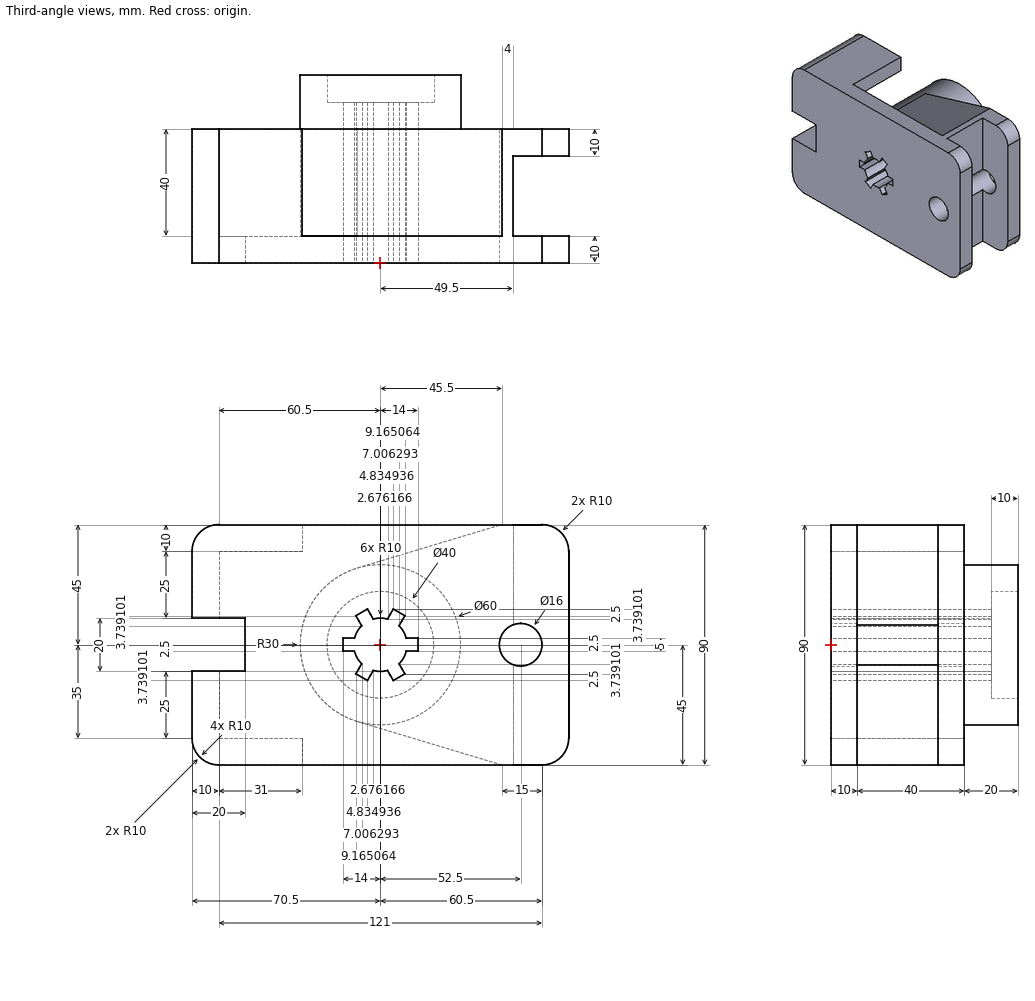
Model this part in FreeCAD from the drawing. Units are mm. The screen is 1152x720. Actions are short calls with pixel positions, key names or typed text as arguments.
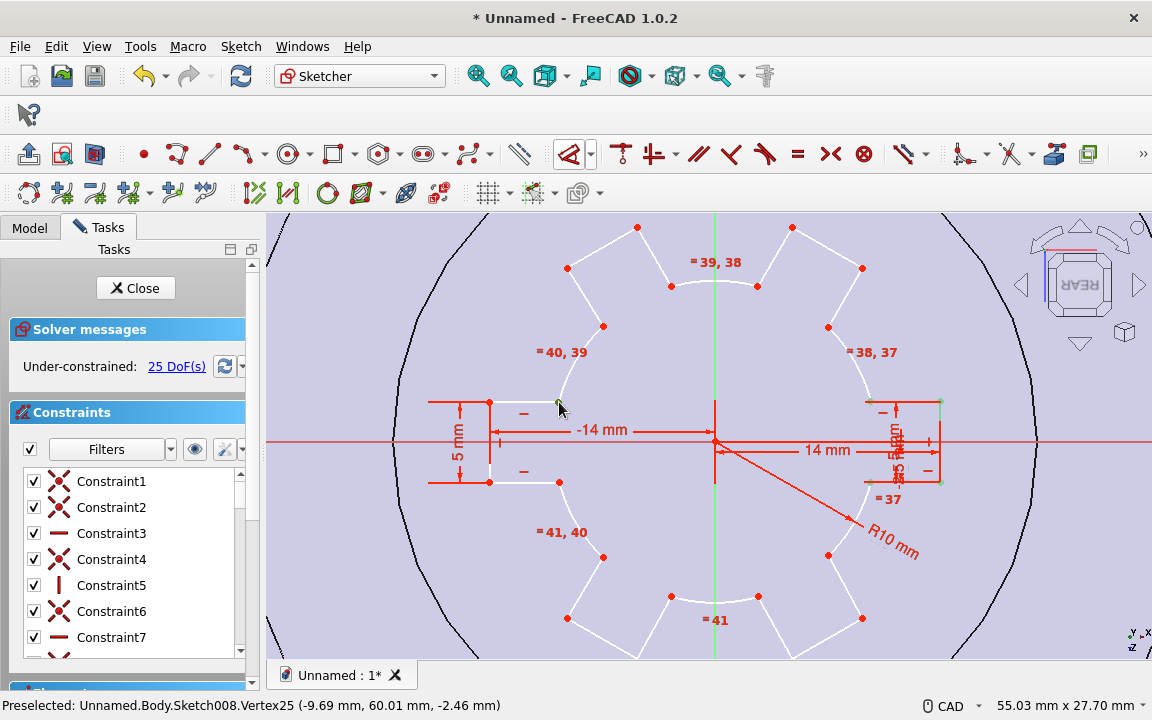
click(590, 154)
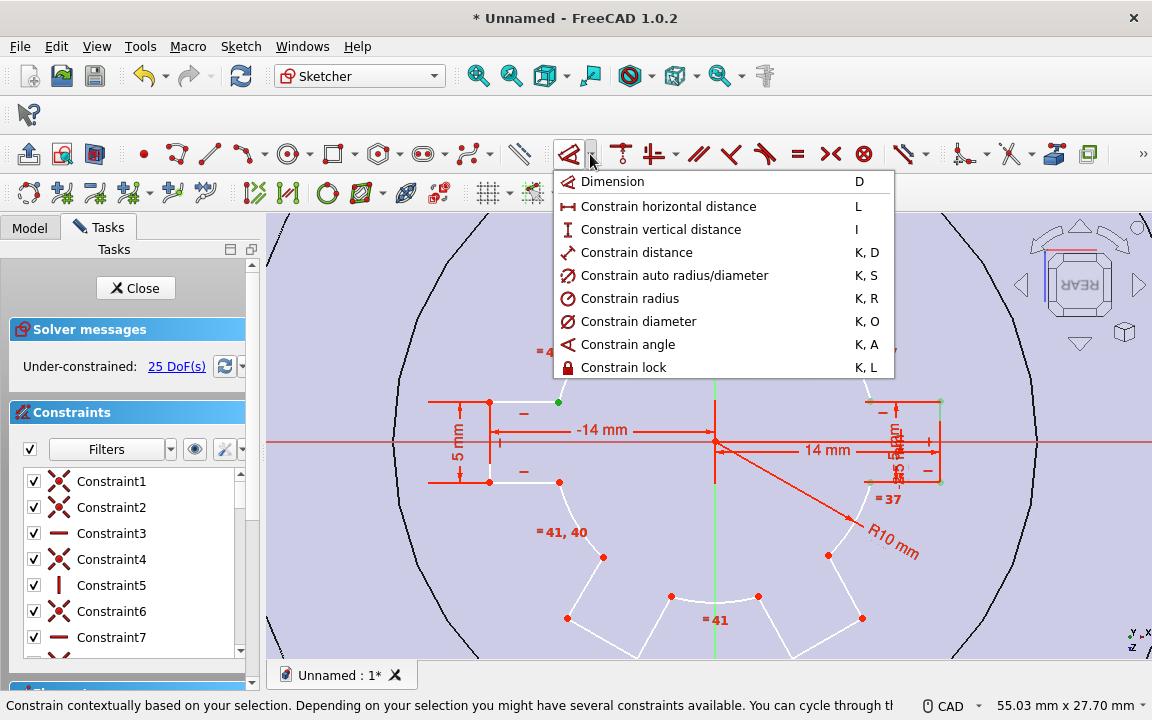
click(724, 230)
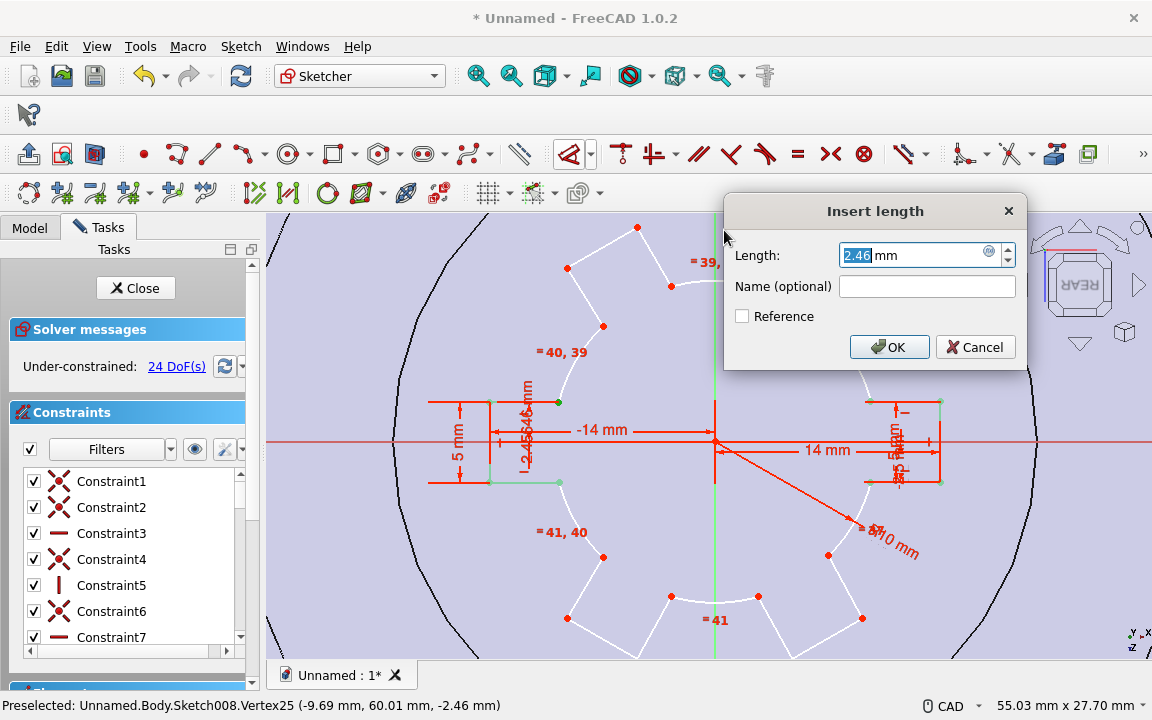
text(2.5)
key(Return)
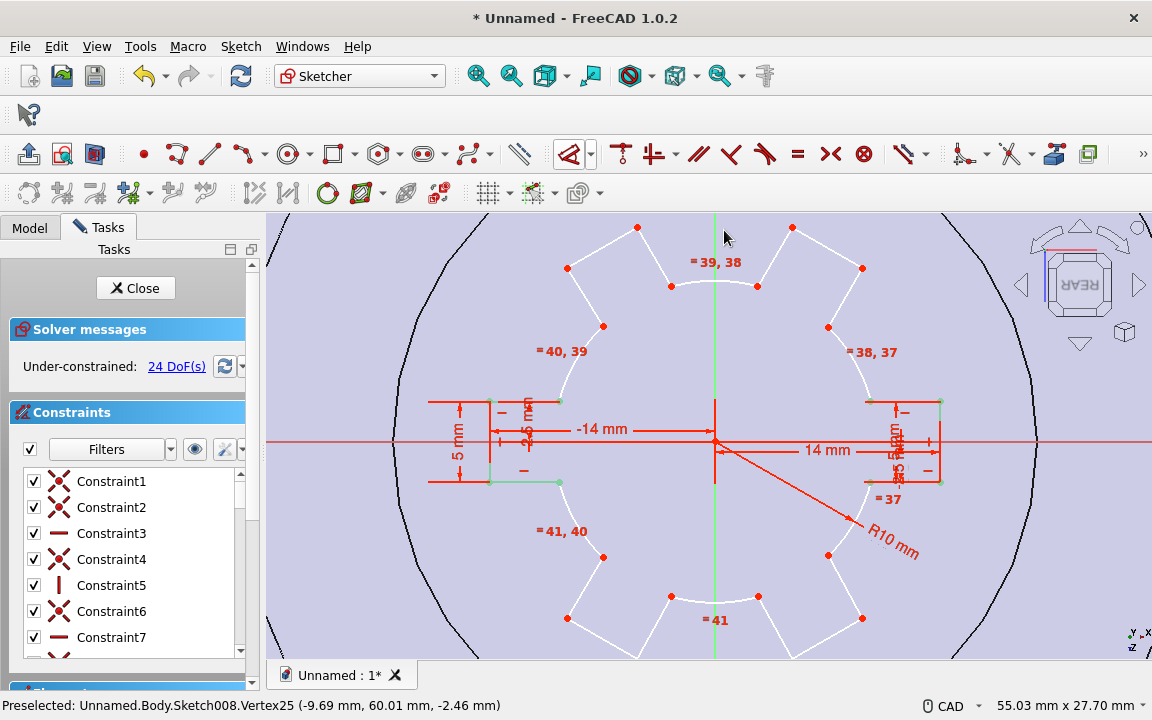
click(841, 631)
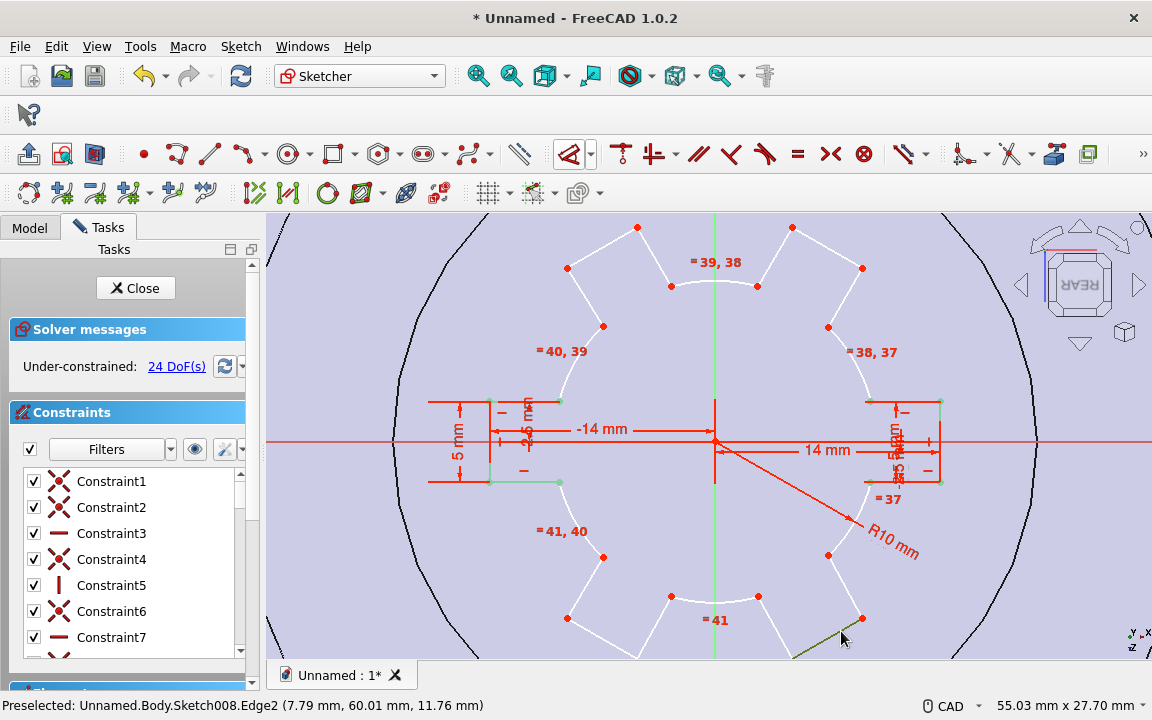
key(i)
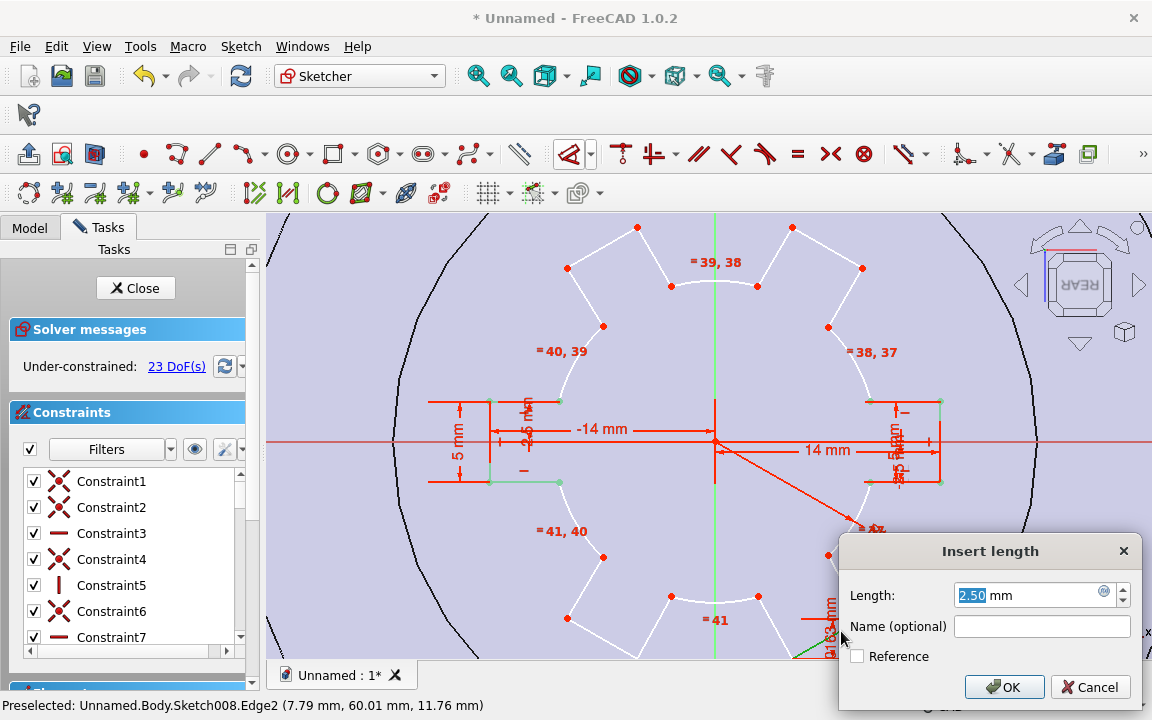
text(2.5)
key(Return)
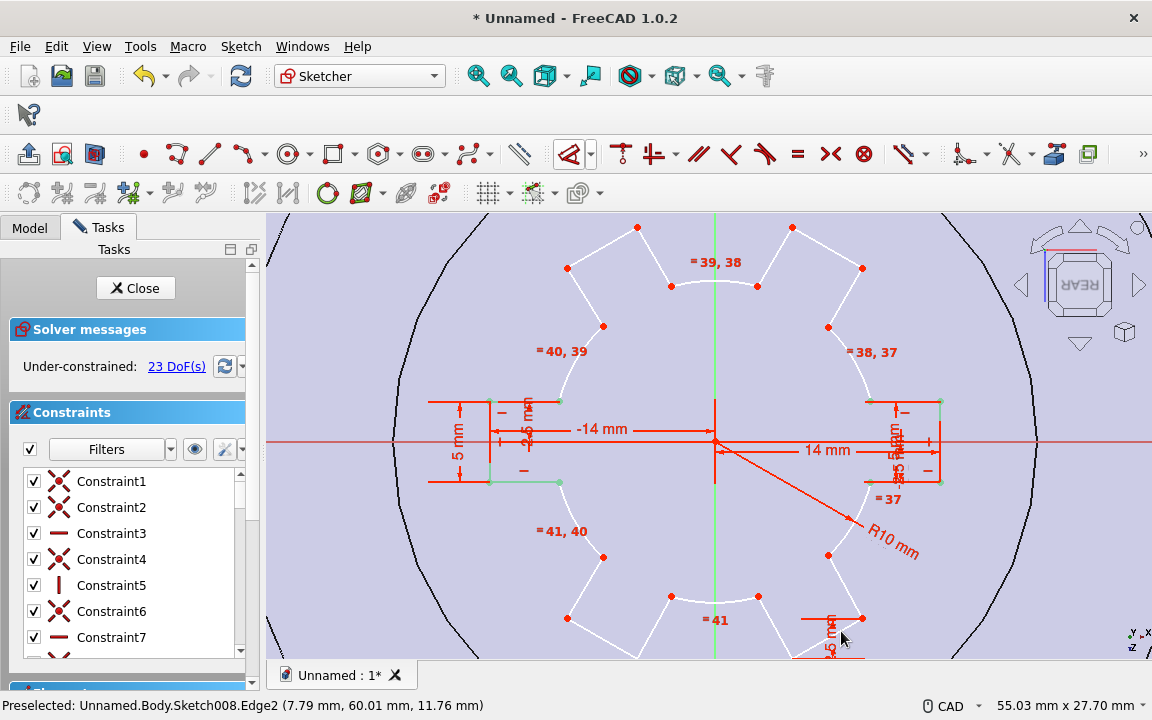
click(841, 256)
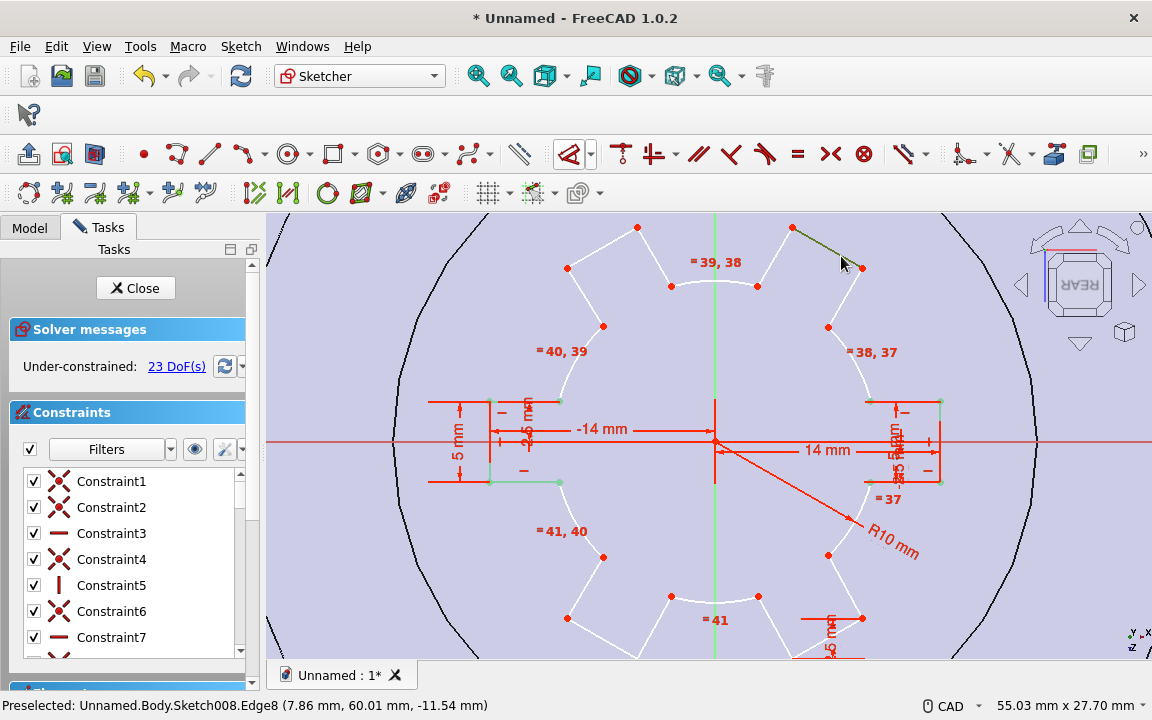
click(590, 154)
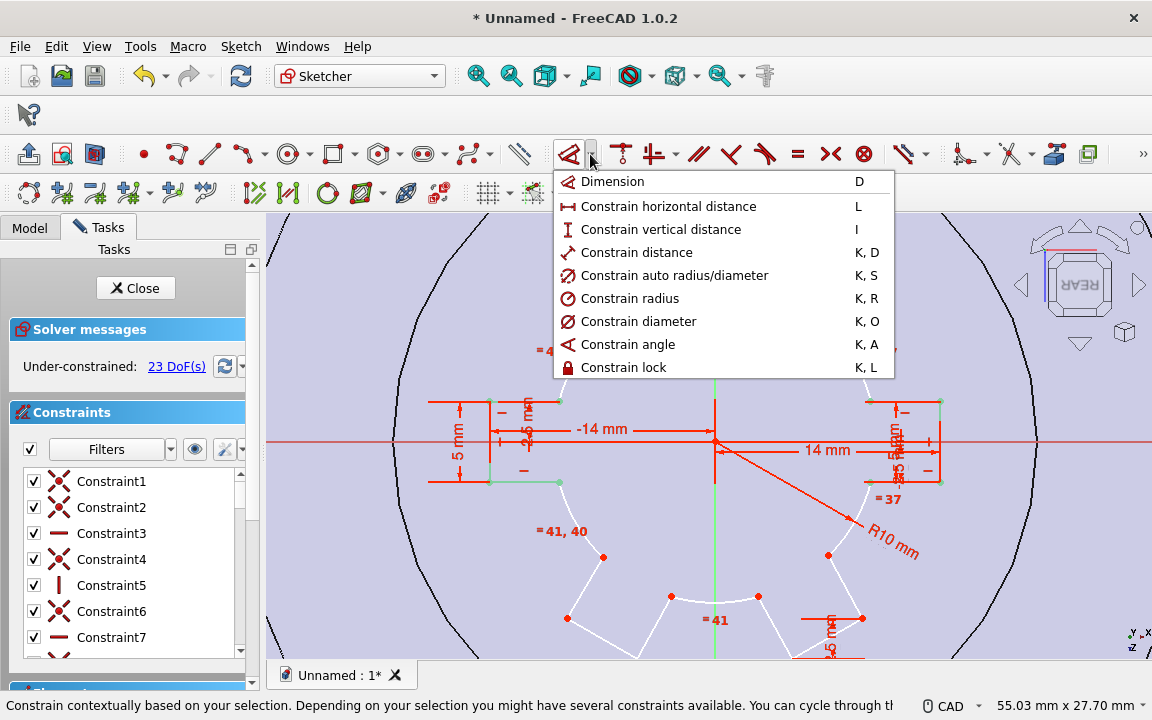
click(724, 230)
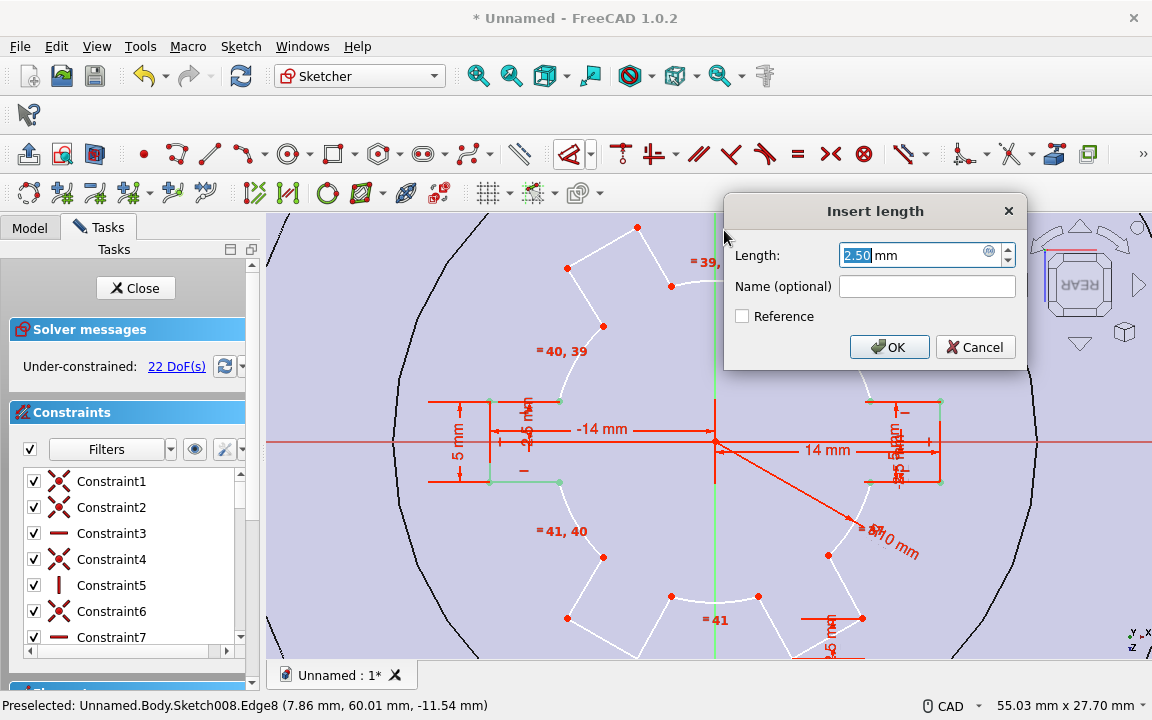
text(2.5)
key(Return)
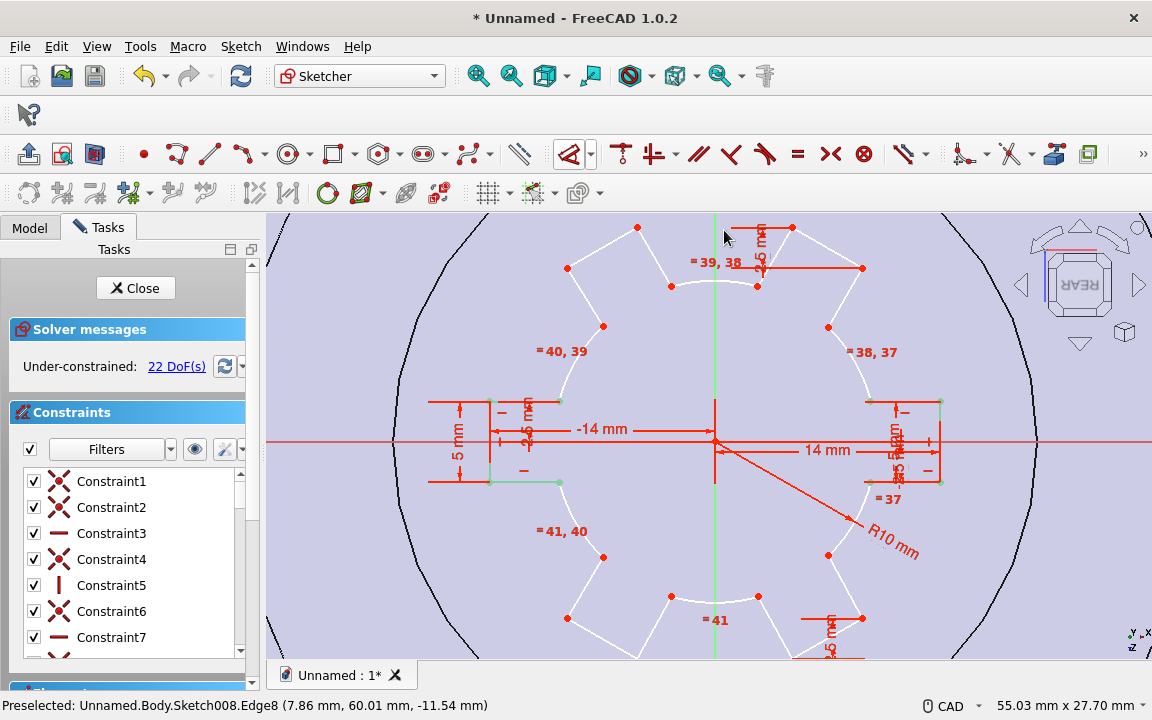
click(588, 256)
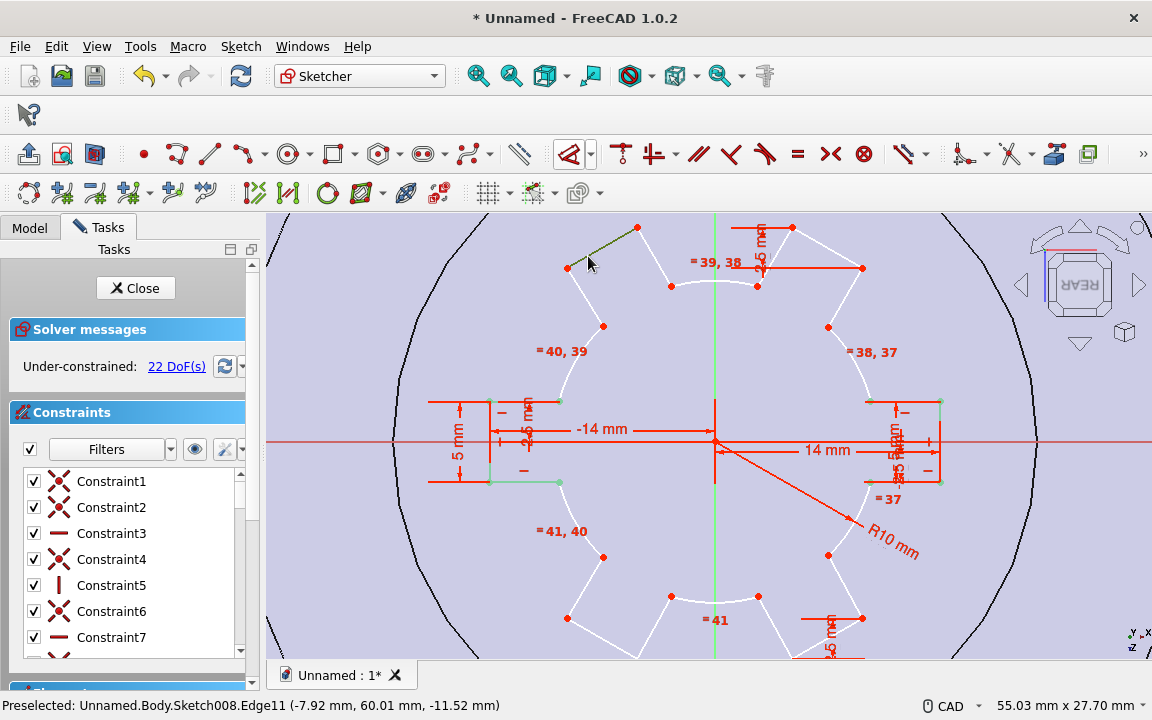
click(590, 154)